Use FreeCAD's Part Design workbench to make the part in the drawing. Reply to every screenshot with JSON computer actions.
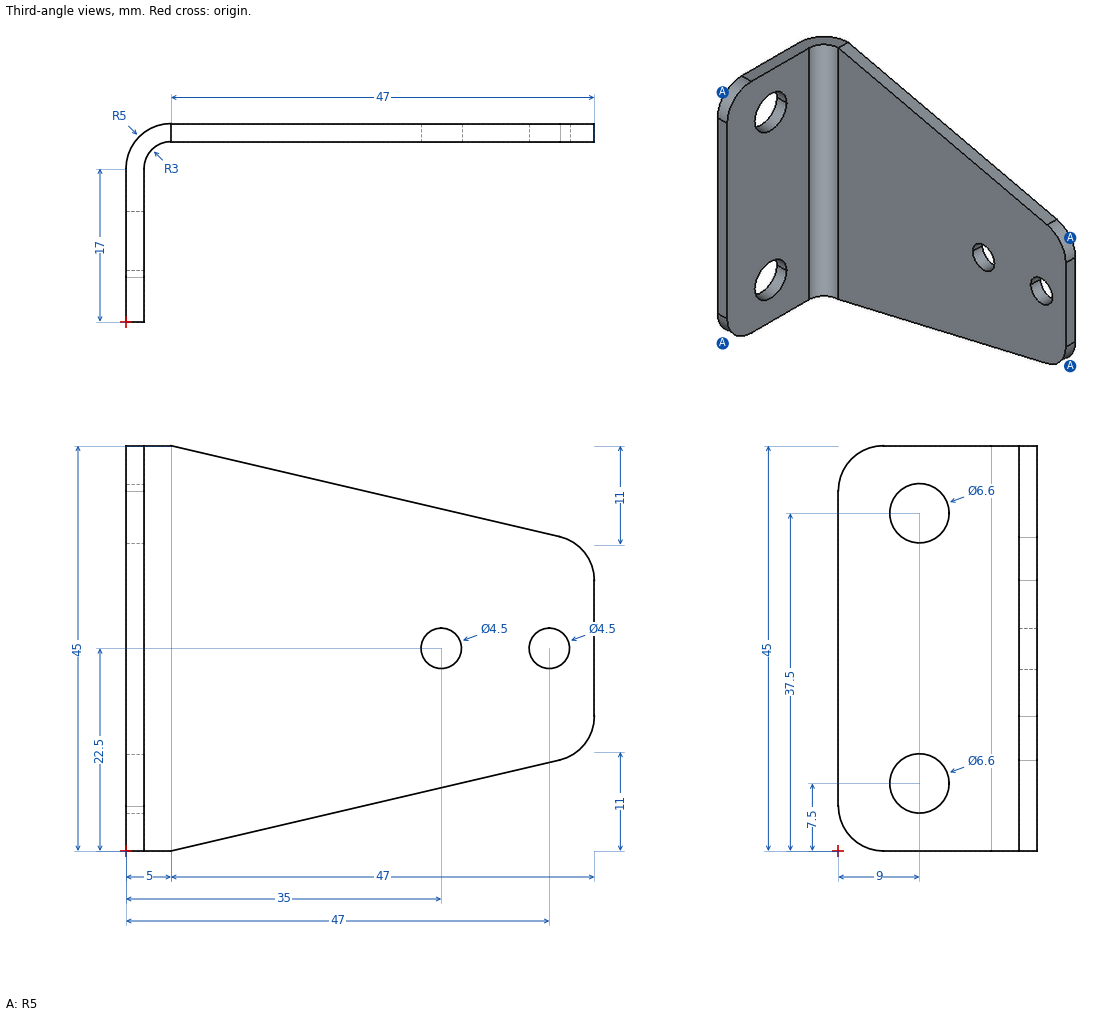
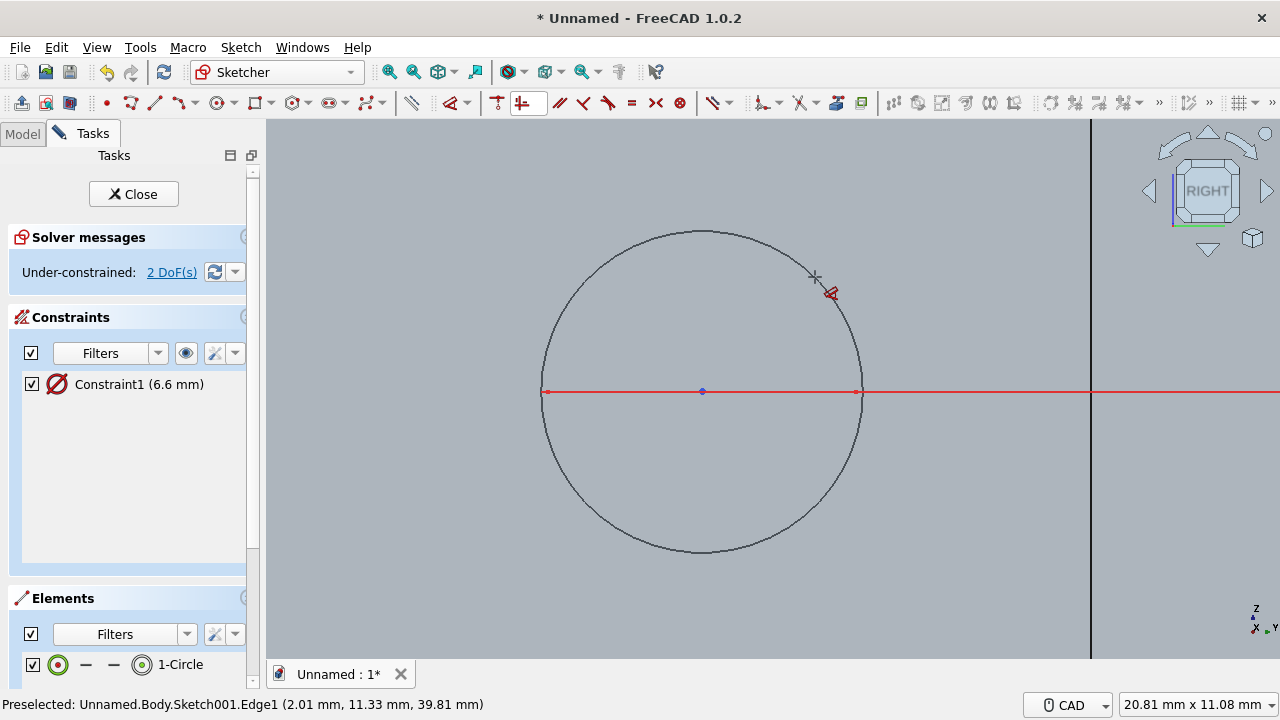
{"action": "left_click", "coordinate": [702, 392]}
{"action": "left_click", "coordinate": [498, 358]}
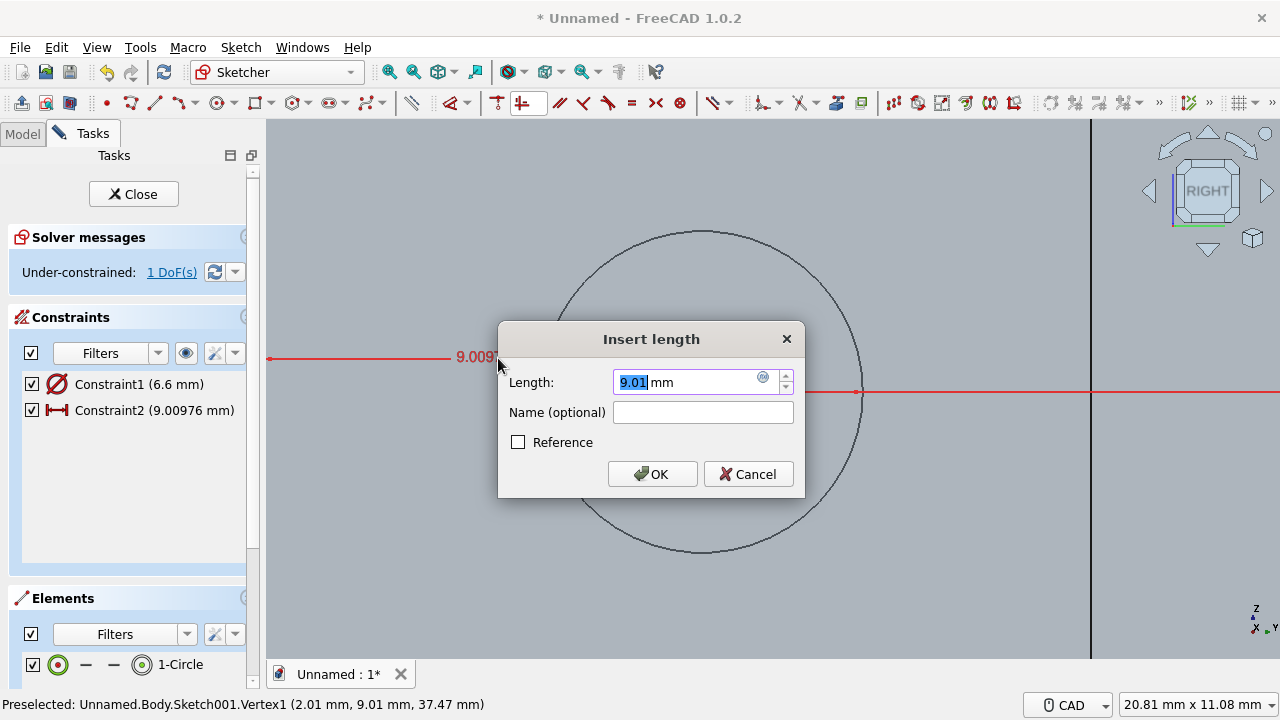
{"action": "type", "text": "9"}
{"action": "key", "text": "Return"}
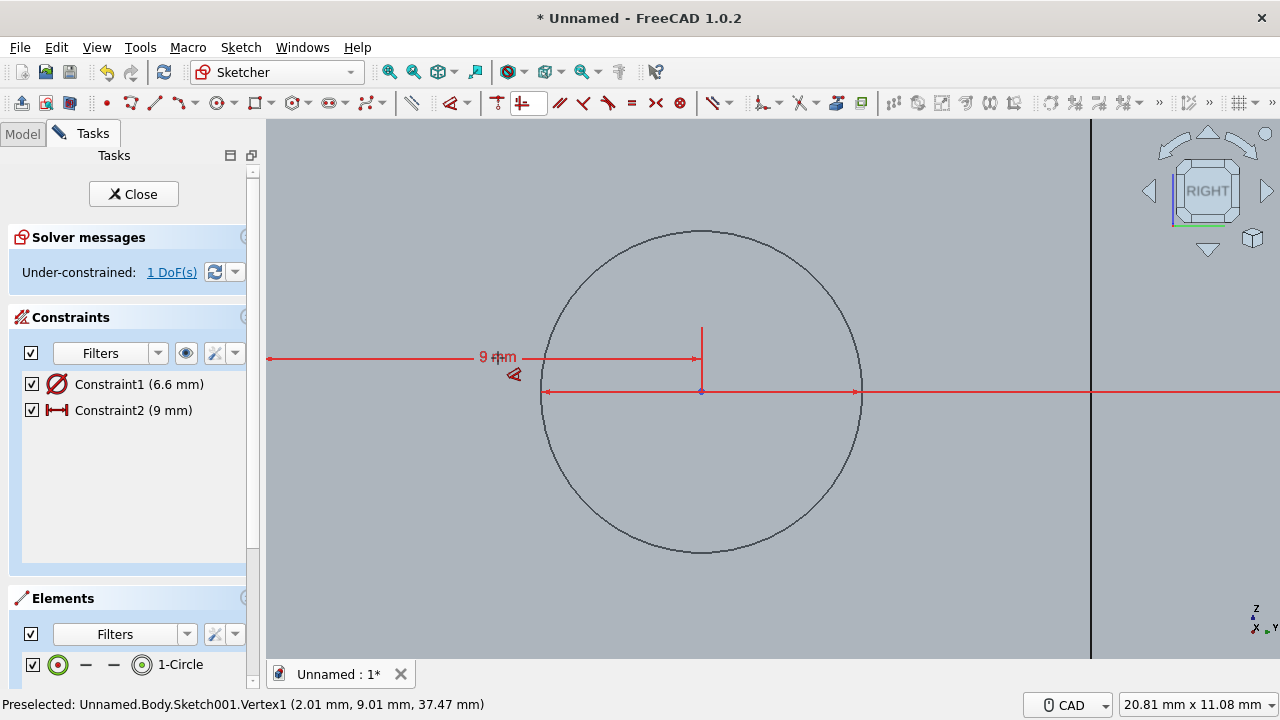
{"action": "left_click", "coordinate": [702, 392]}
{"action": "left_click", "coordinate": [736, 512]}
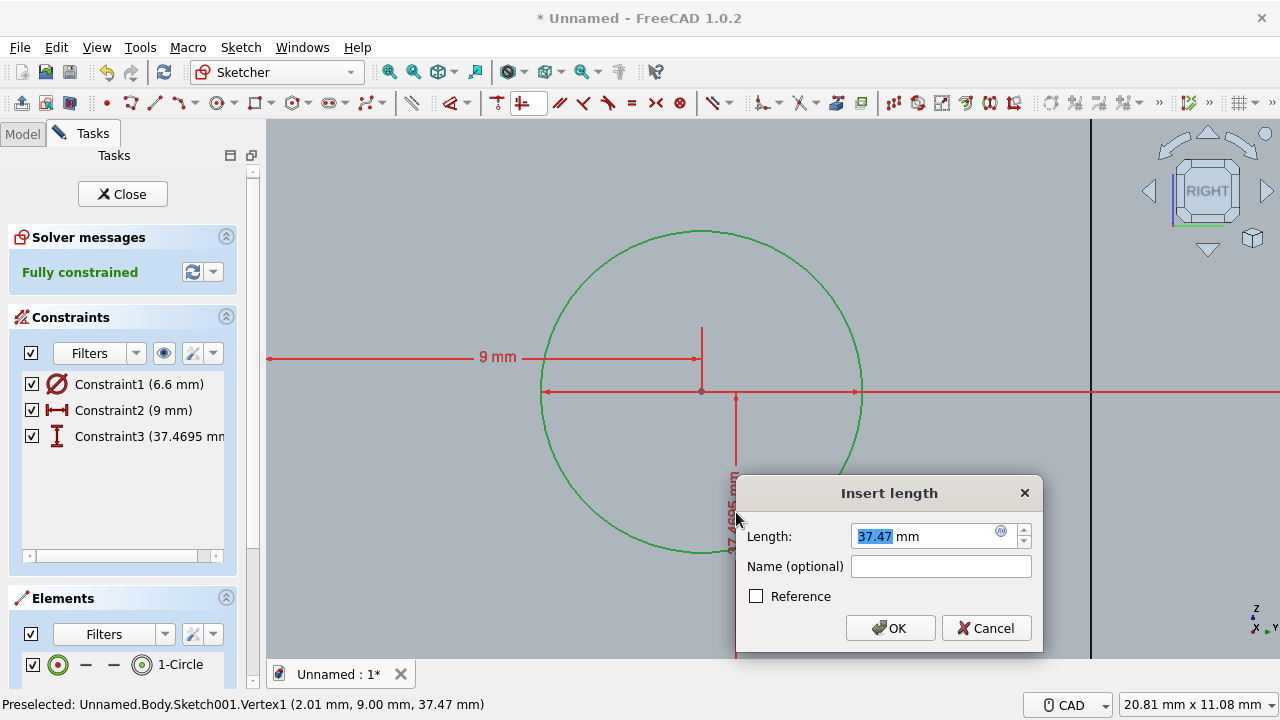
{"action": "type", "text": "37.5"}
{"action": "key", "text": "Return"}
{"action": "key", "text": "Escape"}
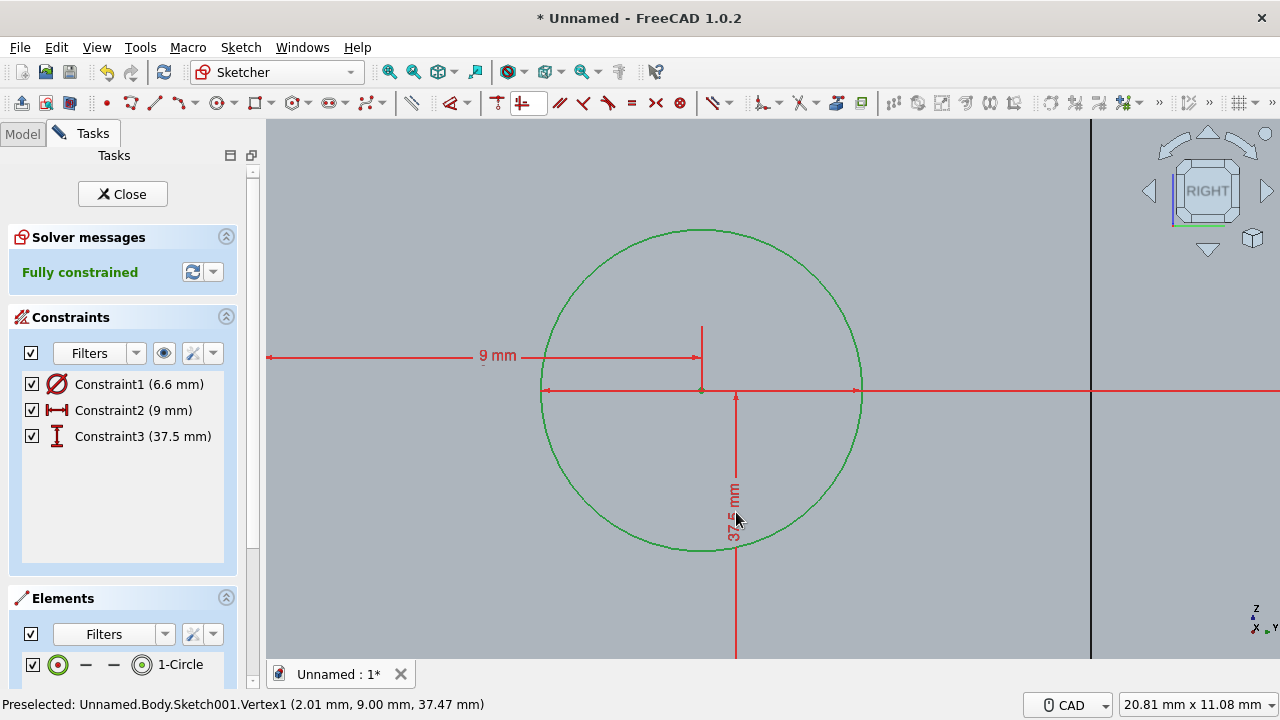
{"action": "left_click", "coordinate": [123, 194]}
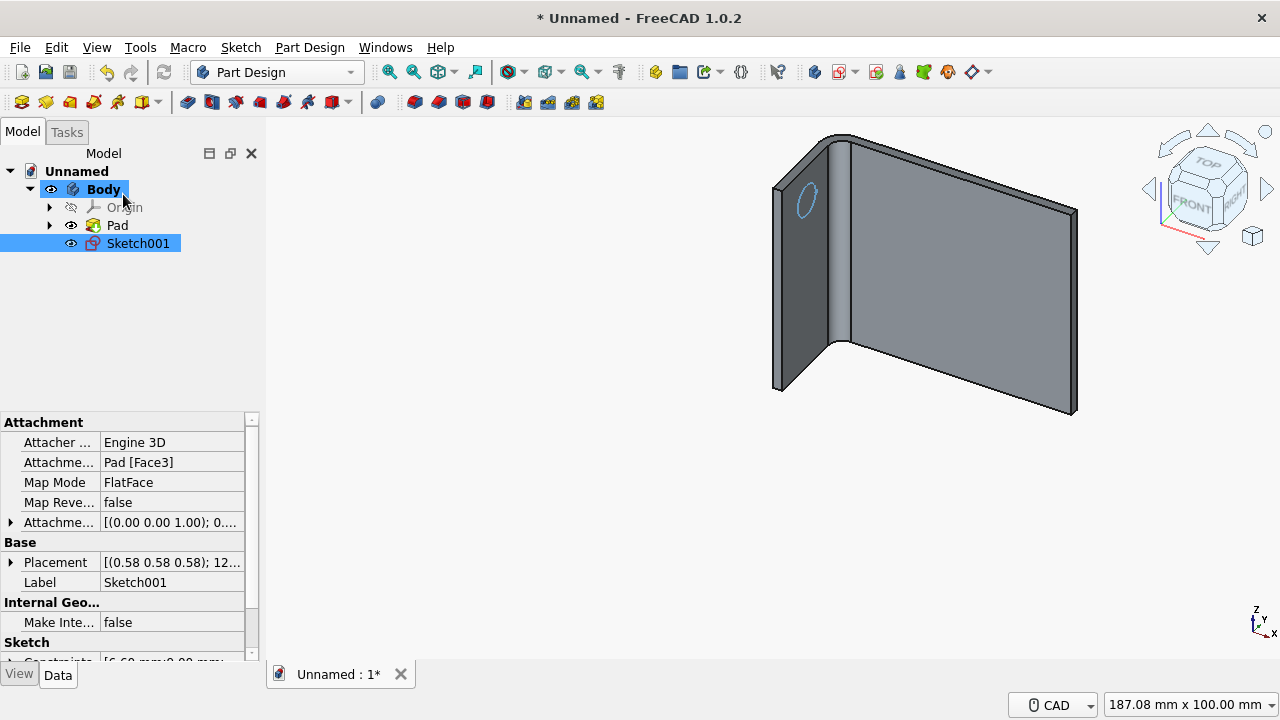
{"action": "left_click", "coordinate": [188, 102]}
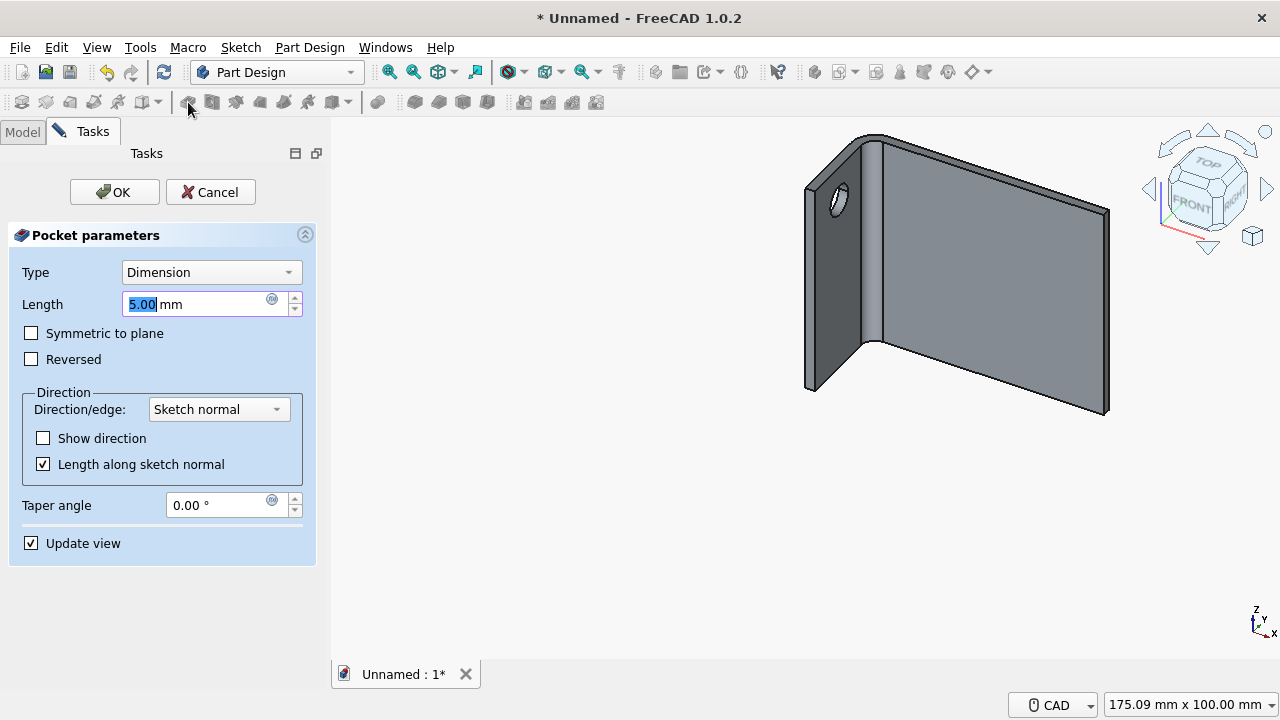
{"action": "left_click", "coordinate": [212, 272]}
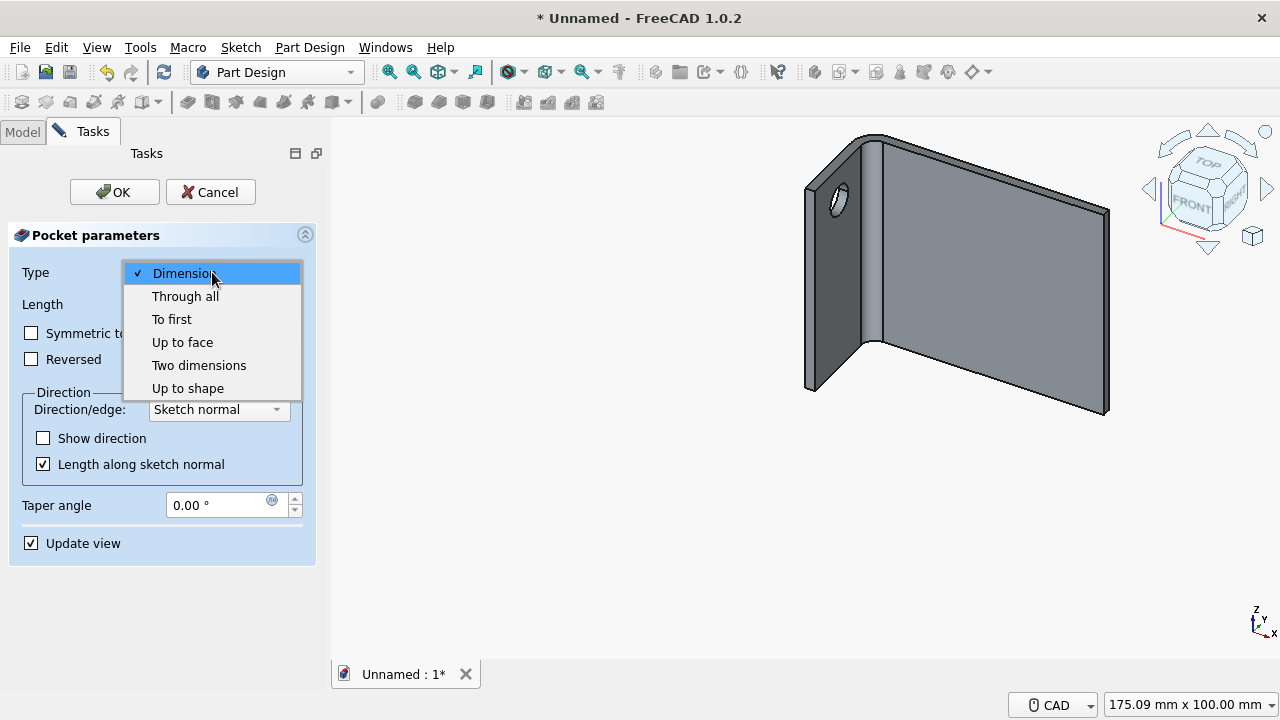
{"action": "left_click", "coordinate": [212, 320]}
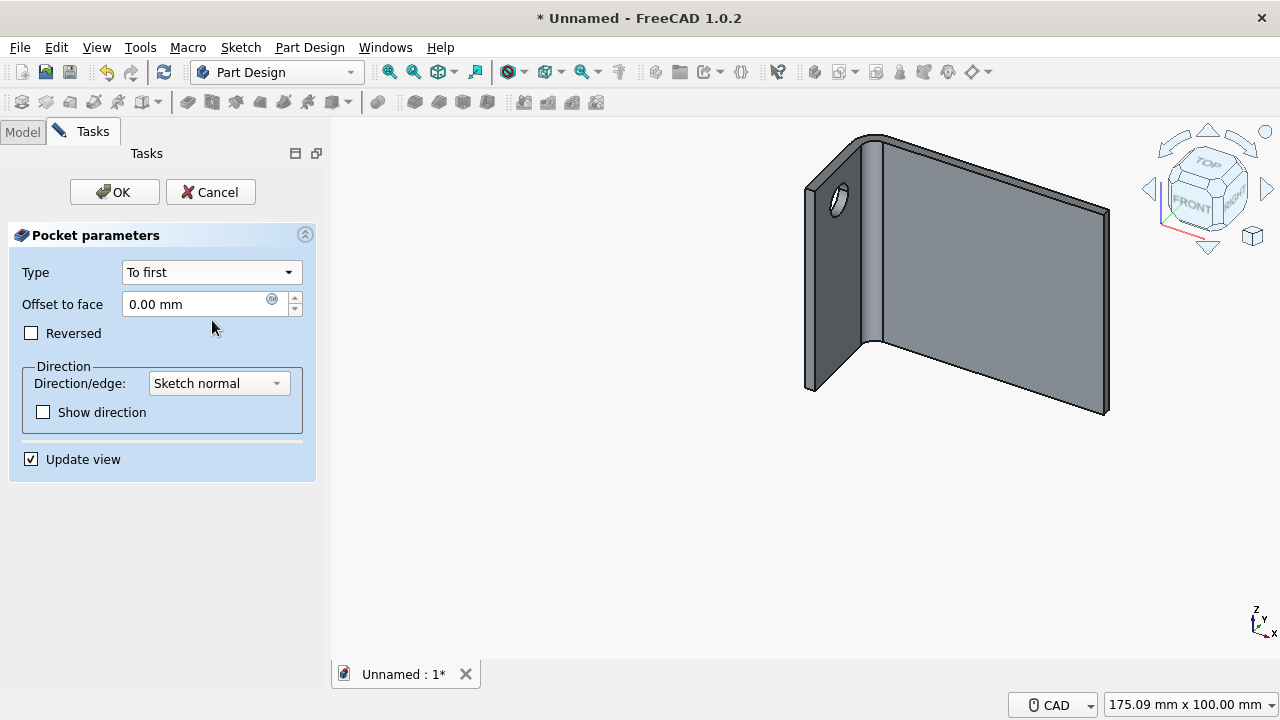
{"action": "left_click", "coordinate": [115, 192]}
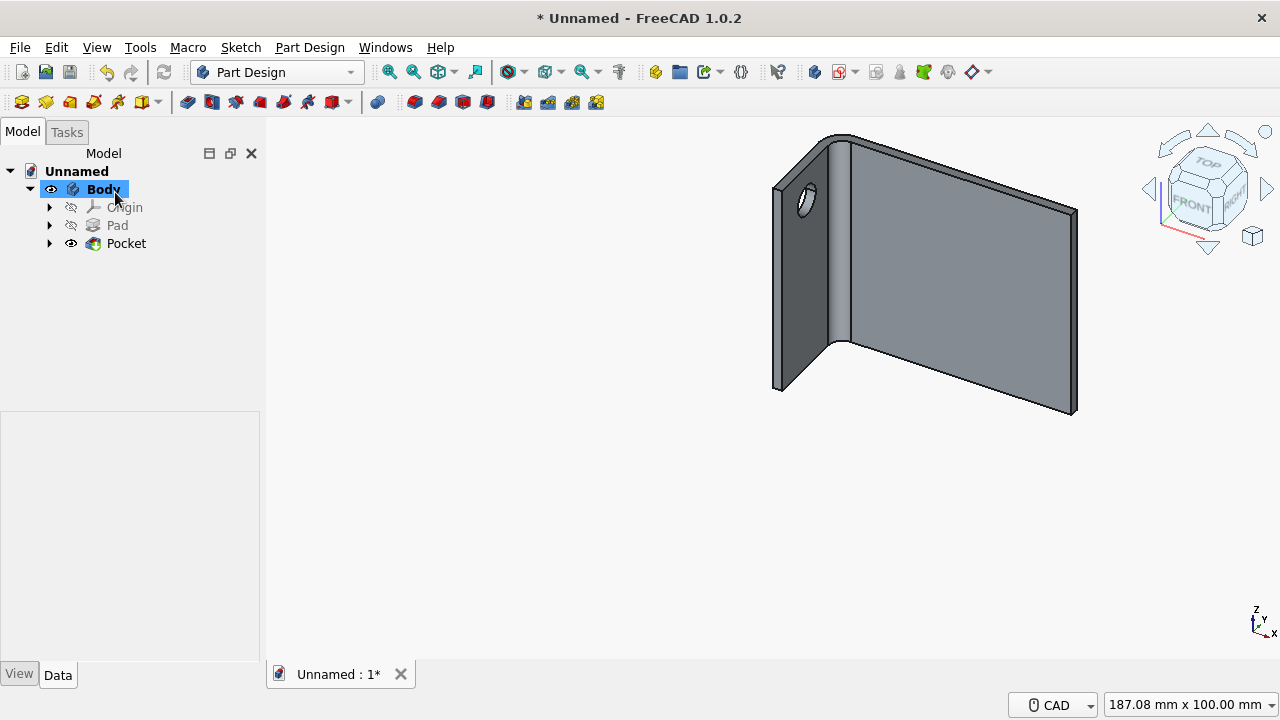
{"action": "left_click", "coordinate": [805, 267]}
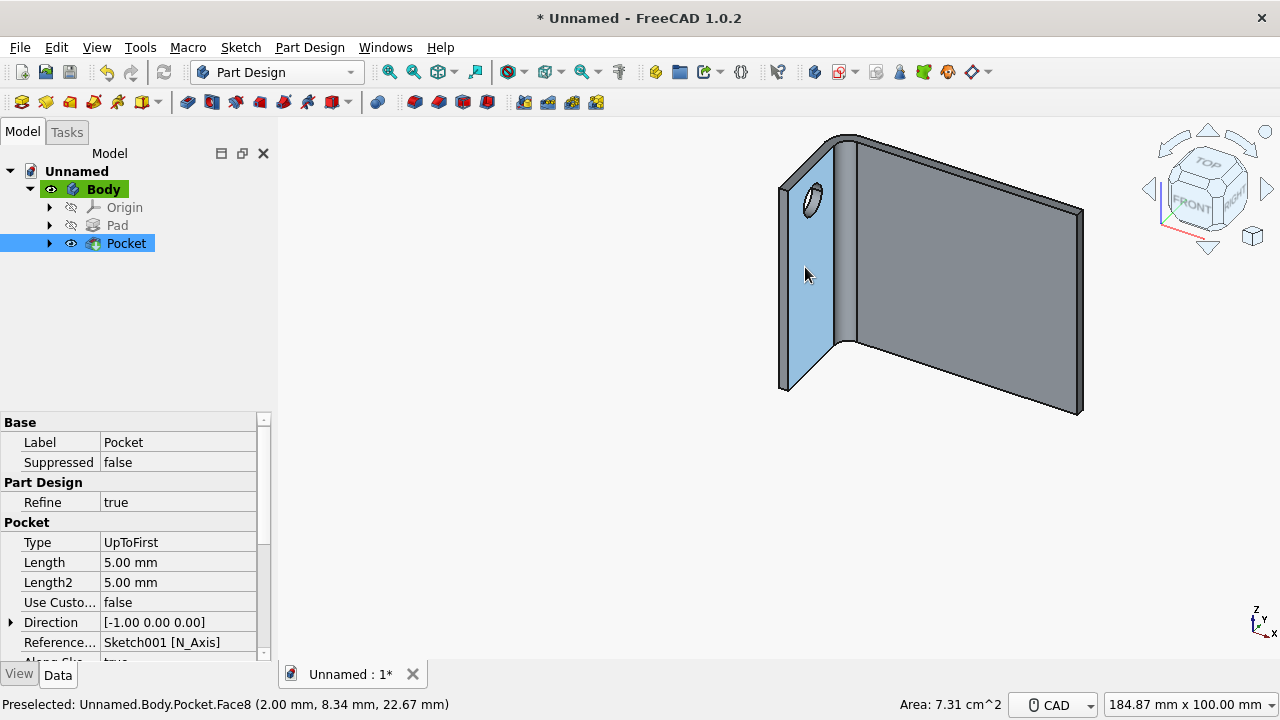
{"action": "left_click", "coordinate": [840, 72]}